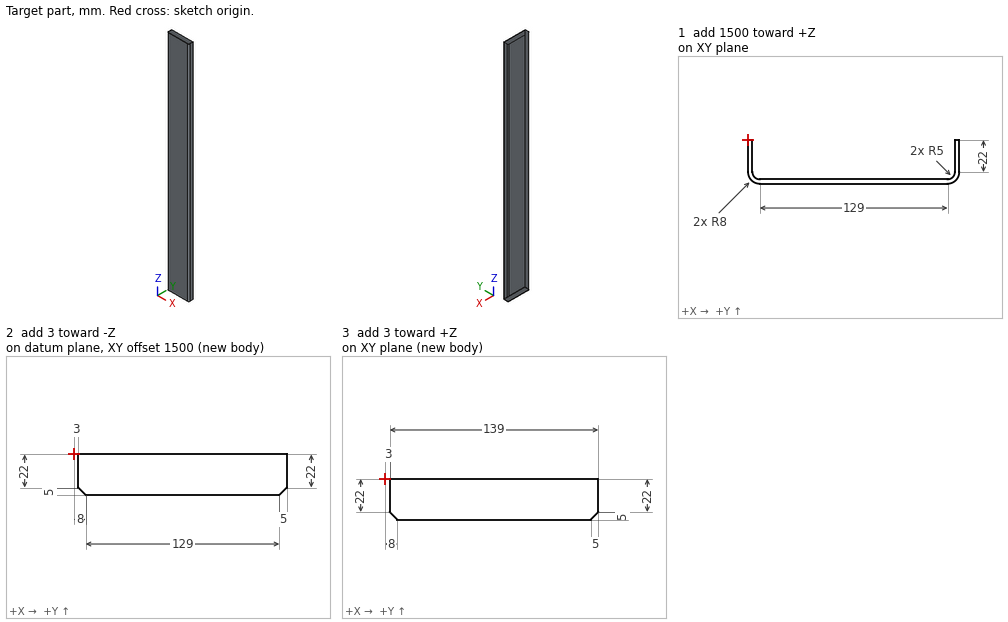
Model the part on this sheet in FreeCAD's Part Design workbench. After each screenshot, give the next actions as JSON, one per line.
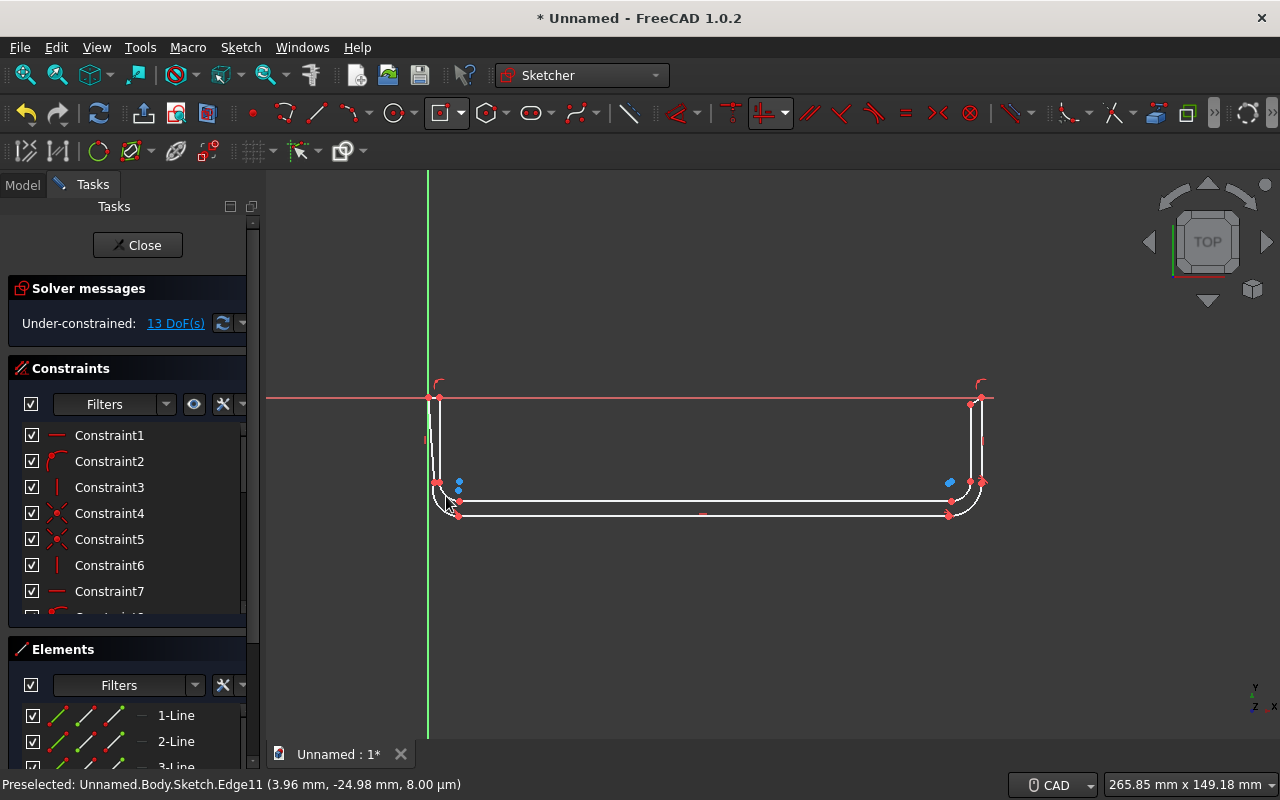
{"action": "scroll", "coordinate": [440, 423], "scroll_direction": "up", "scroll_amount": 2}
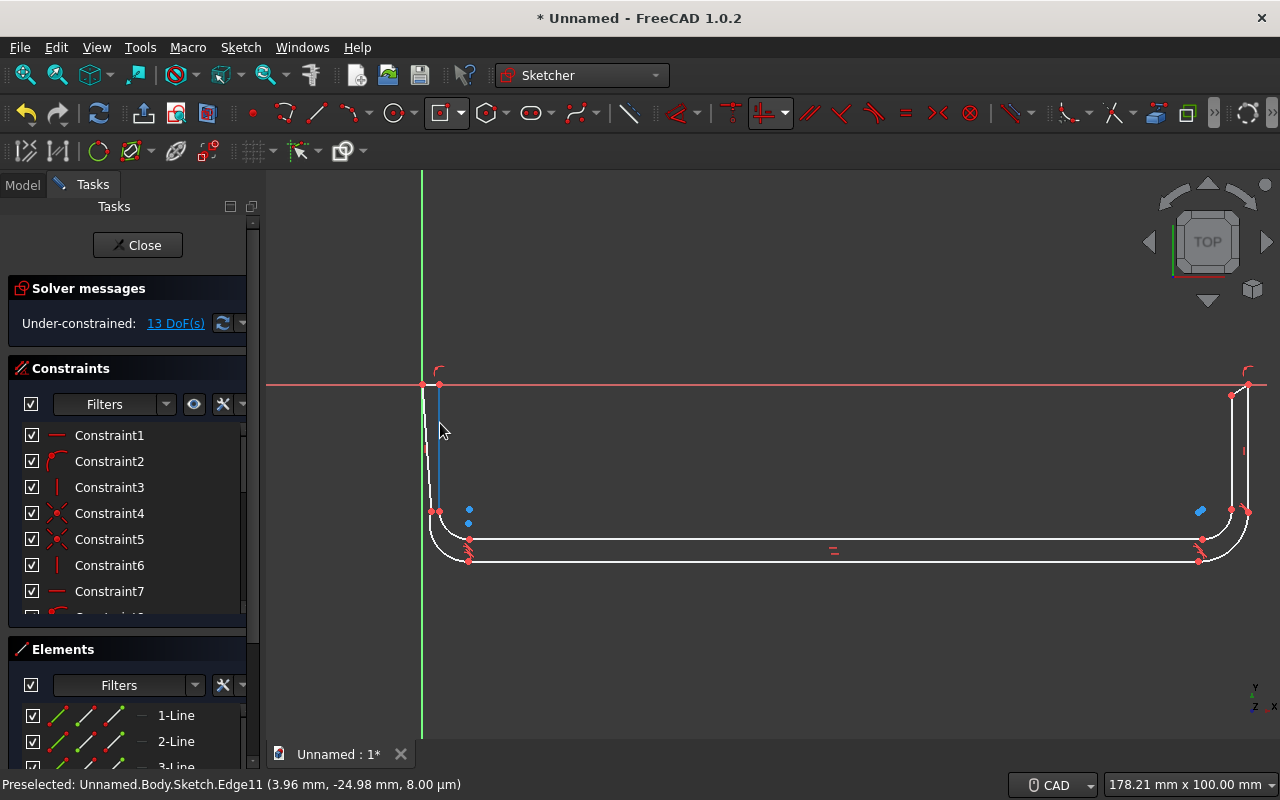
{"action": "left_click", "coordinate": [439, 423]}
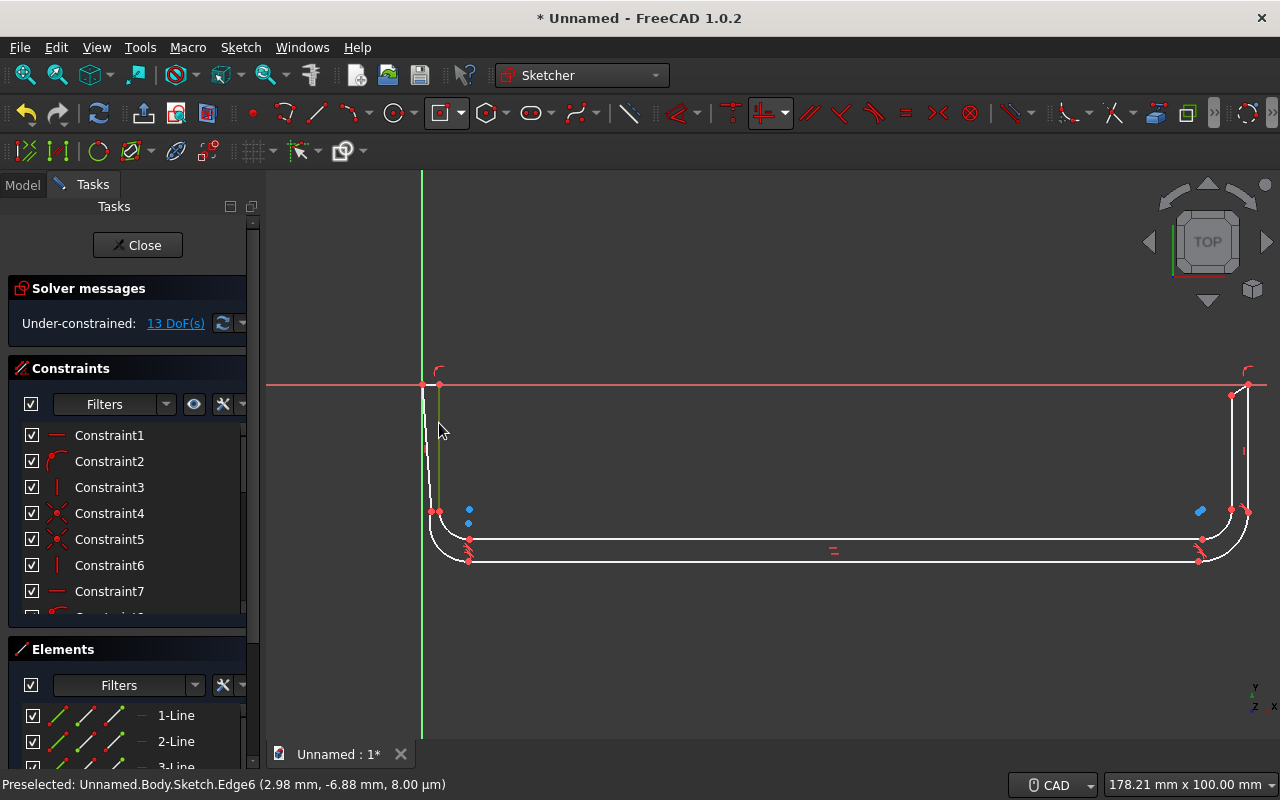
{"action": "left_click", "coordinate": [443, 524]}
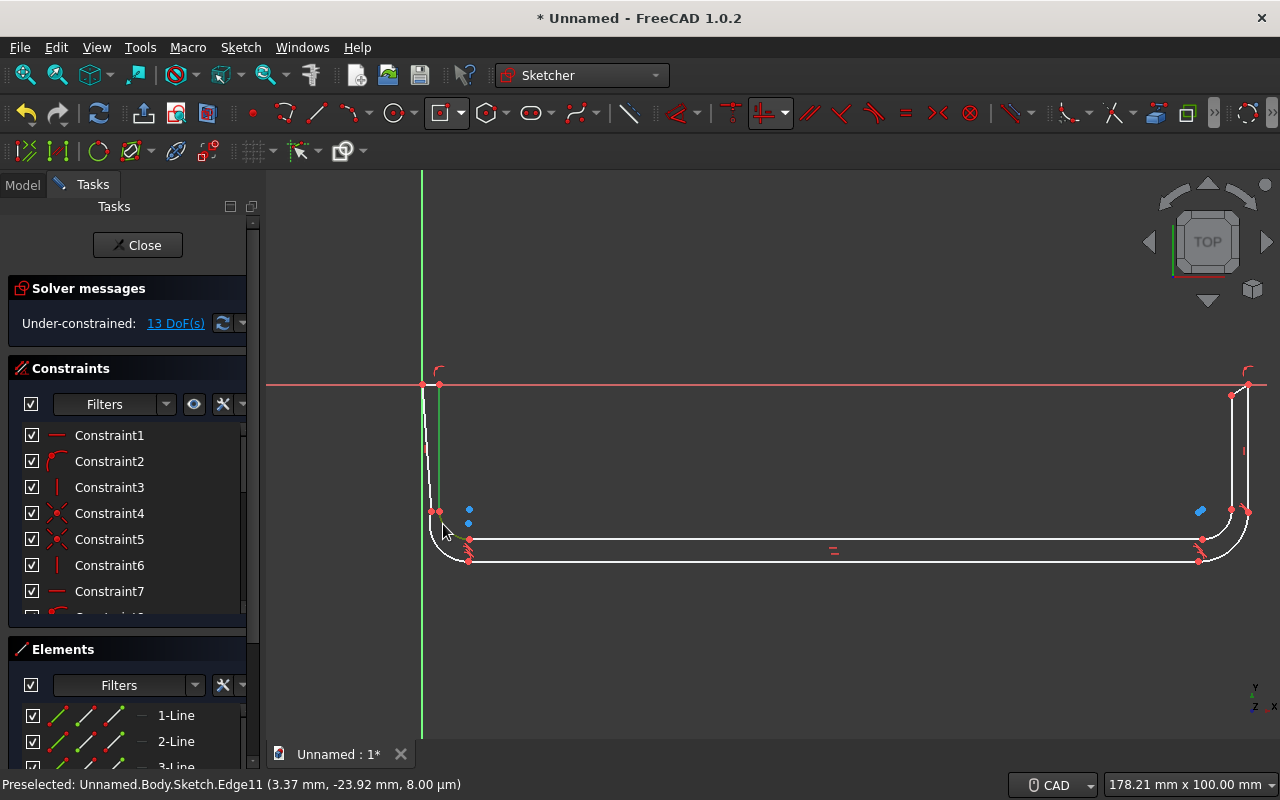
{"action": "key", "text": "t"}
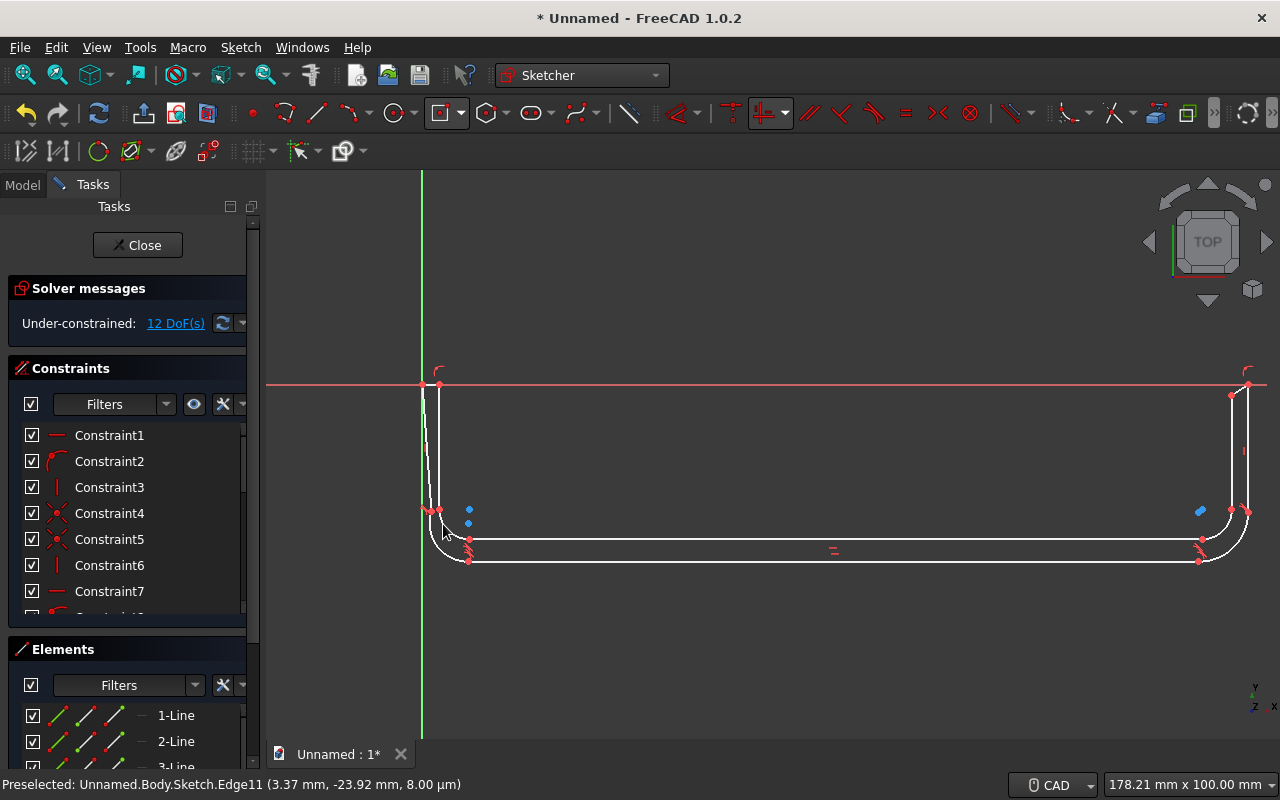
{"action": "left_click", "coordinate": [425, 423]}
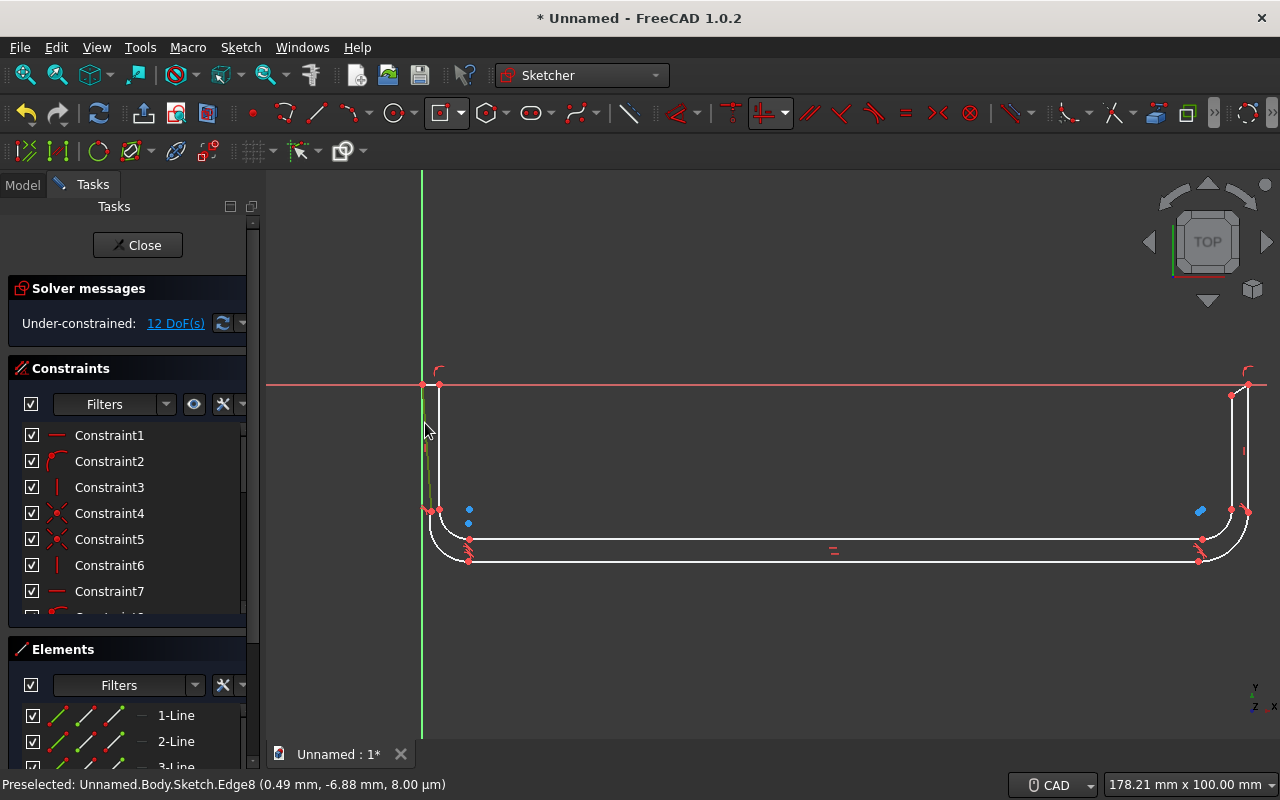
{"action": "left_click", "coordinate": [448, 556]}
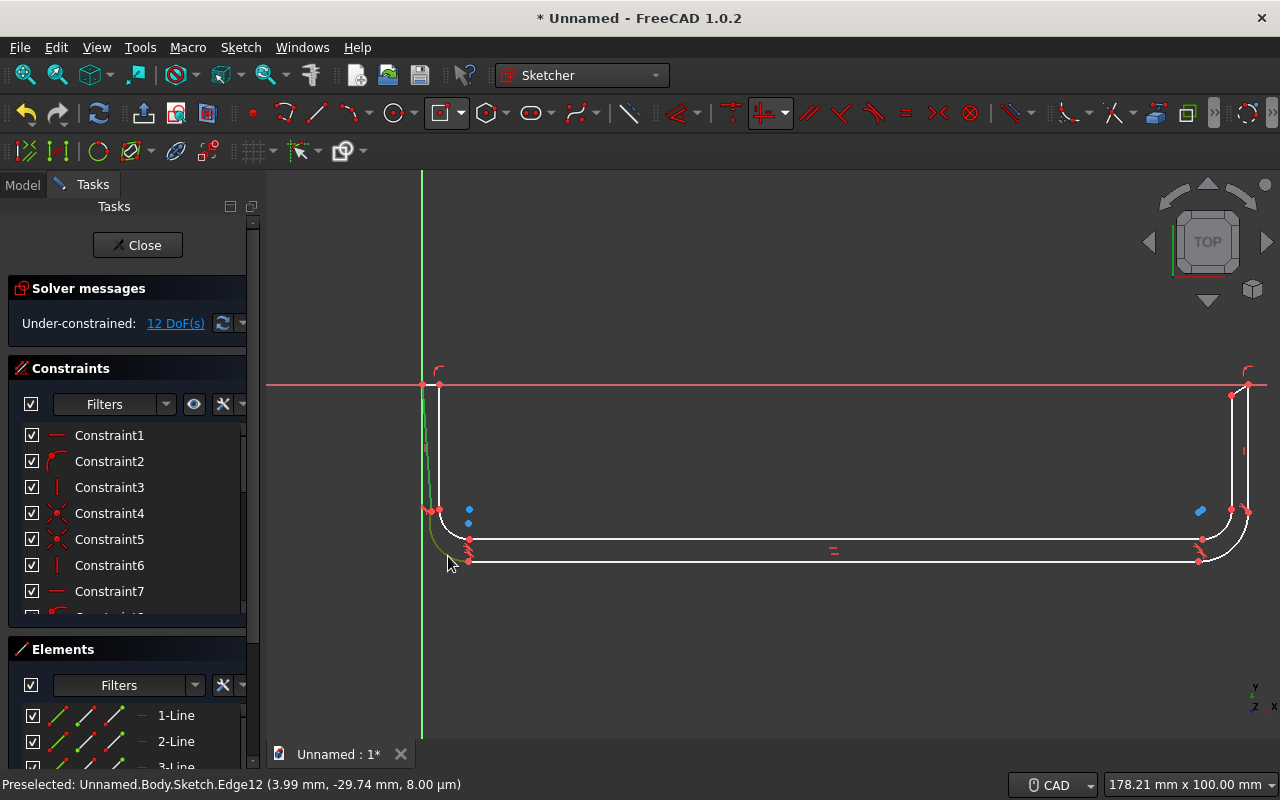
{"action": "key", "text": "t"}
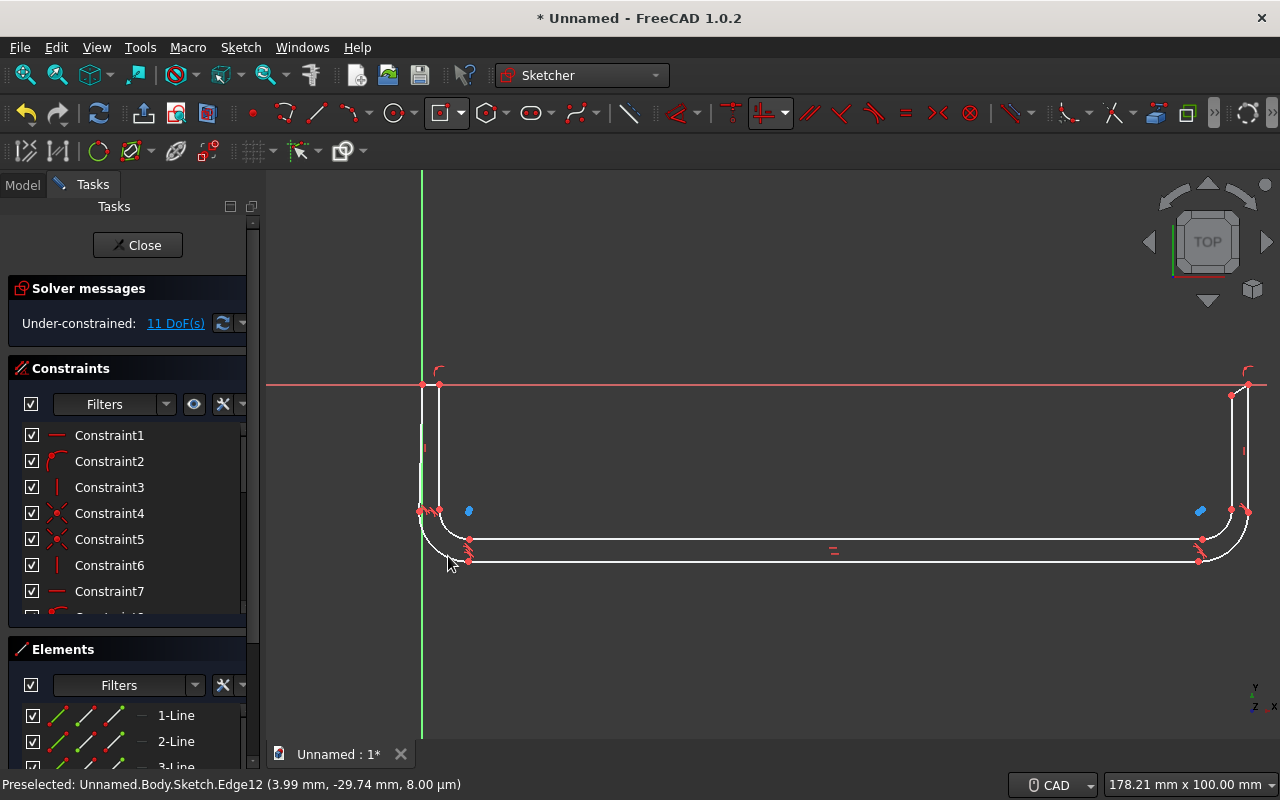
{"action": "scroll", "coordinate": [439, 423], "scroll_direction": "down", "scroll_amount": 2}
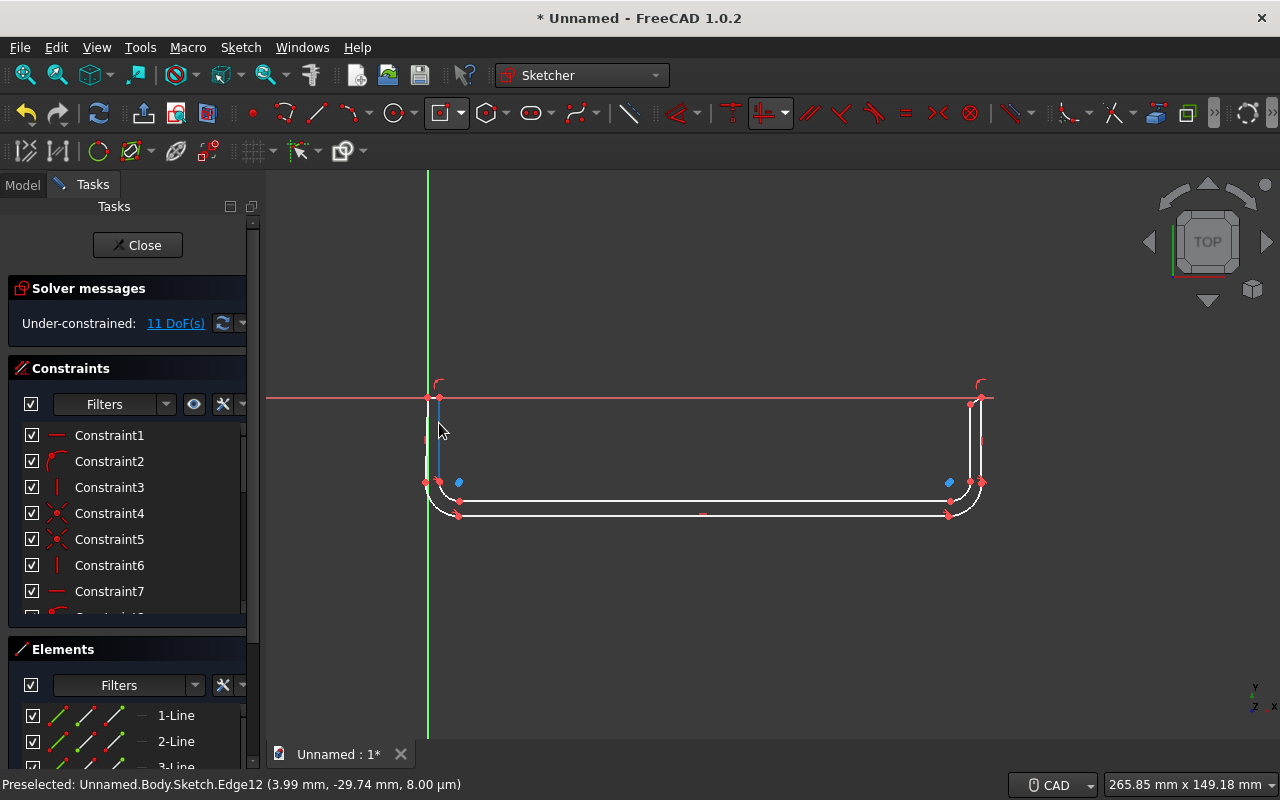
{"action": "scroll", "coordinate": [975, 402], "scroll_direction": "up", "scroll_amount": 6}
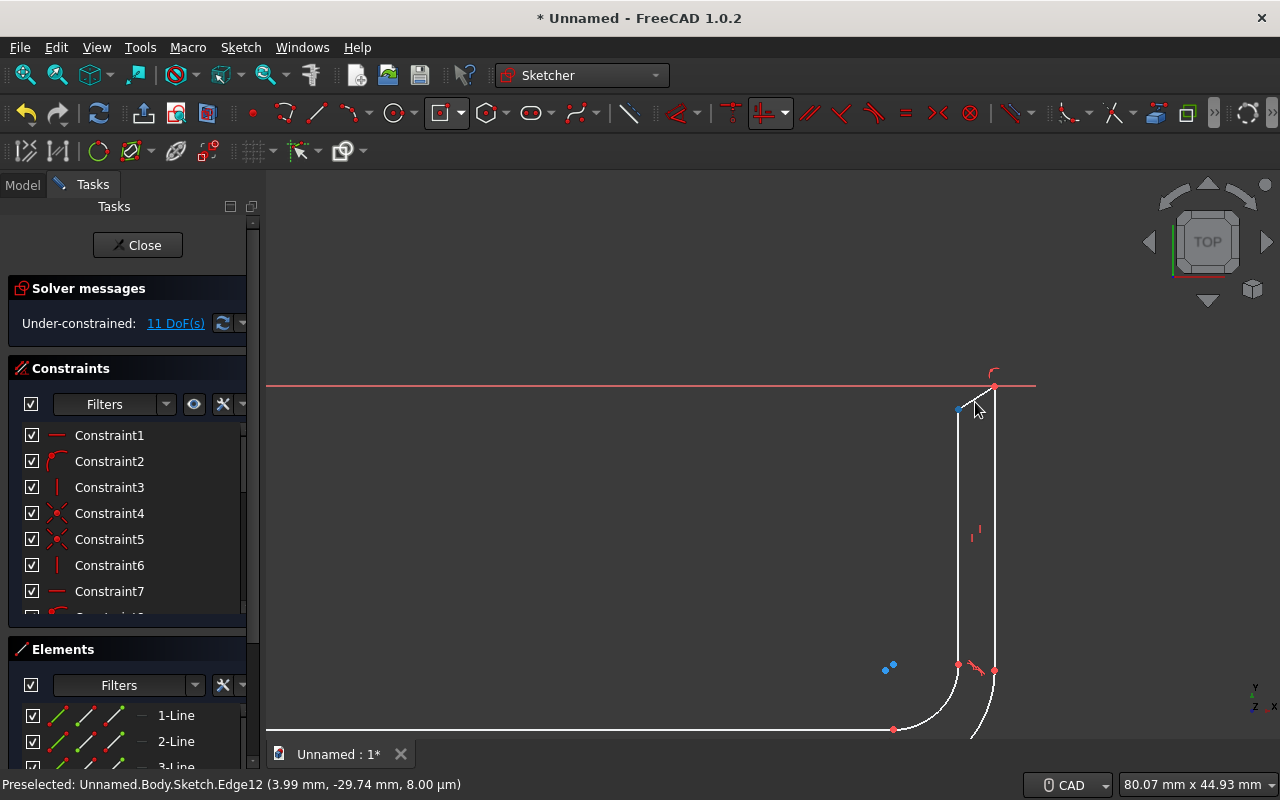
{"action": "left_click", "coordinate": [973, 400]}